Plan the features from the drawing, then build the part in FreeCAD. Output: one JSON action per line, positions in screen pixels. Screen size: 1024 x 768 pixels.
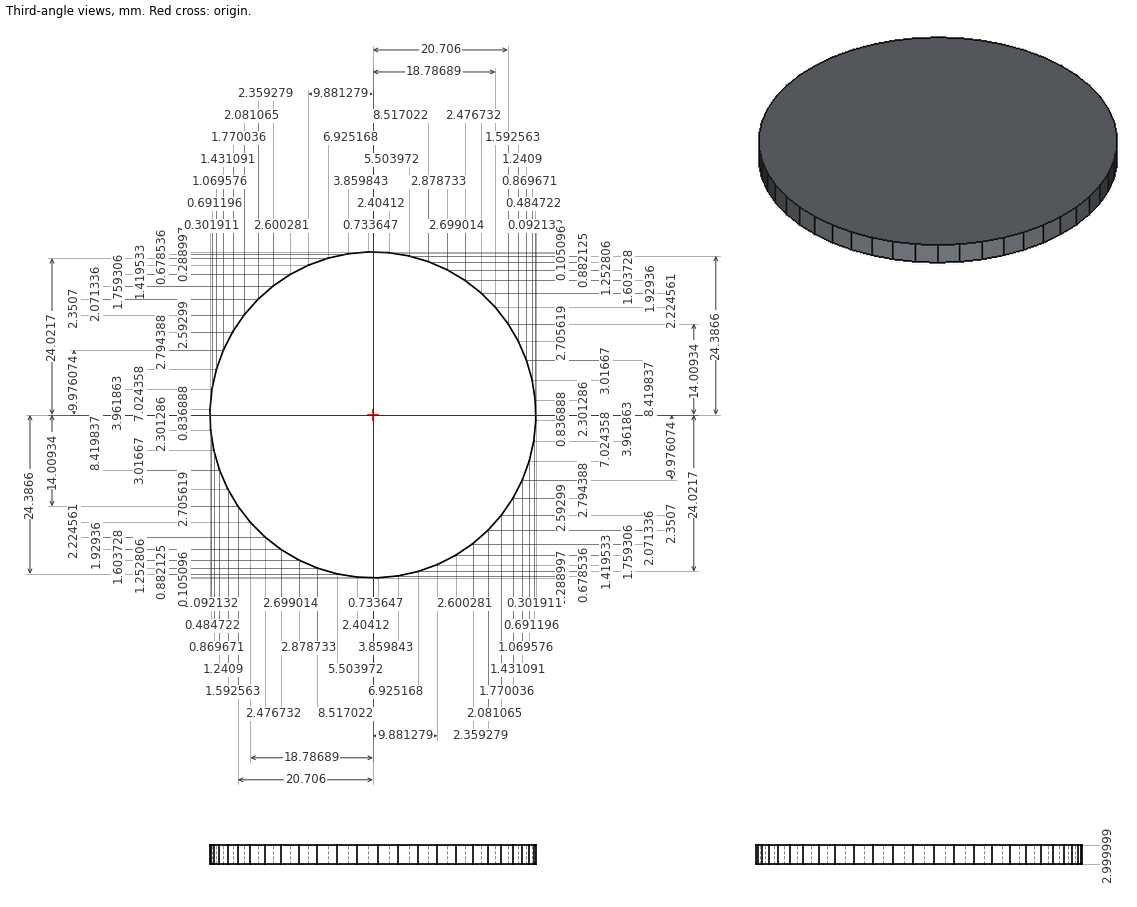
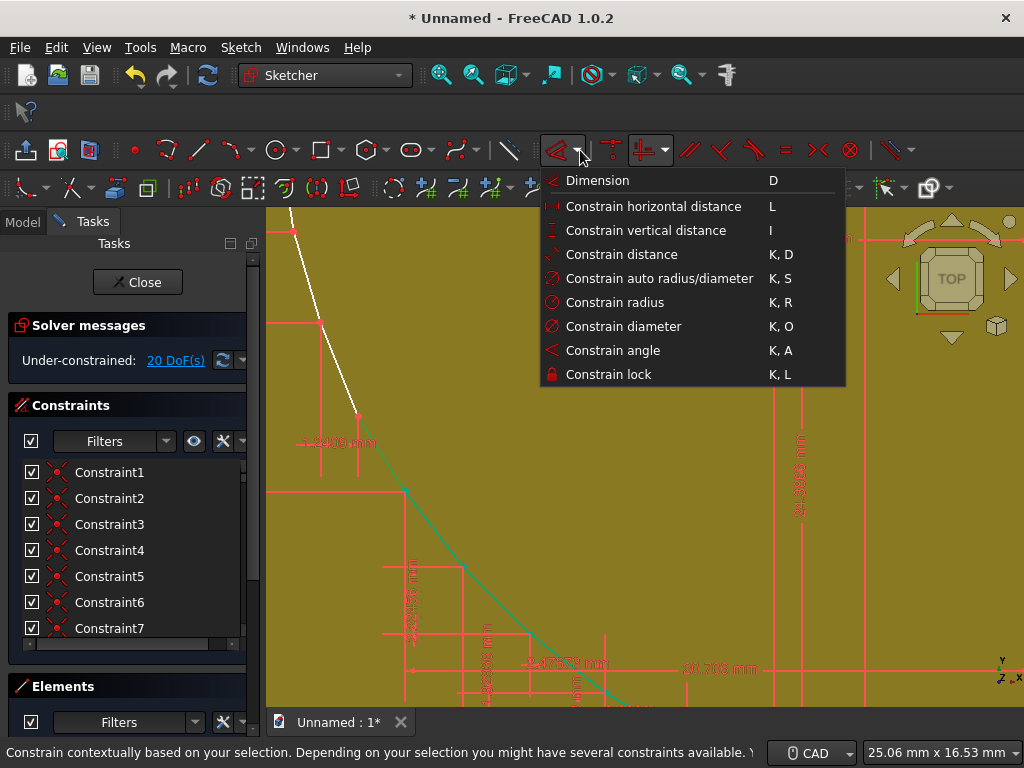
{"action": "left_click", "coordinate": [693, 206]}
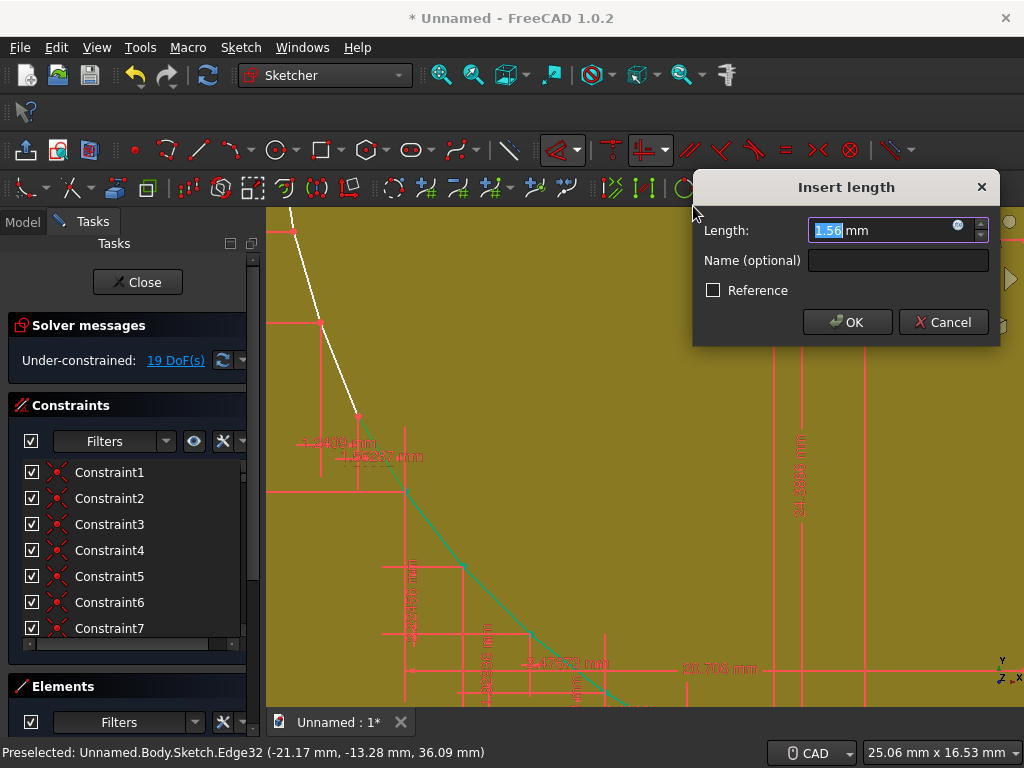
{"action": "type", "text": "1.592563"}
{"action": "key", "text": "Return"}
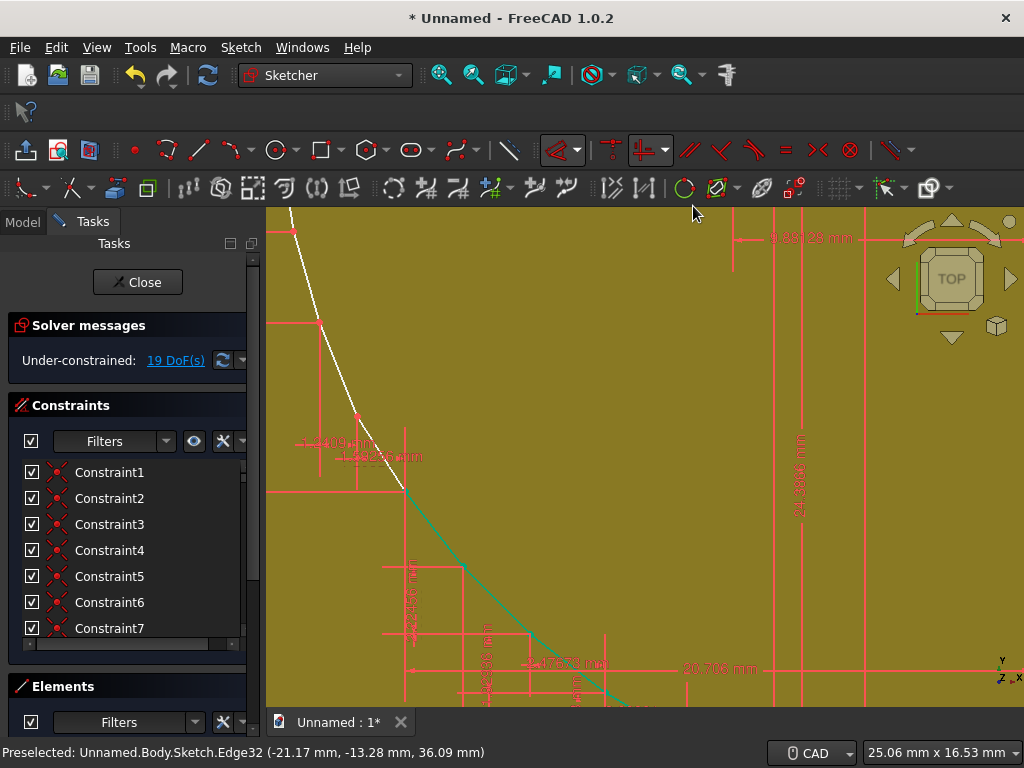
{"action": "left_click", "coordinate": [391, 469]}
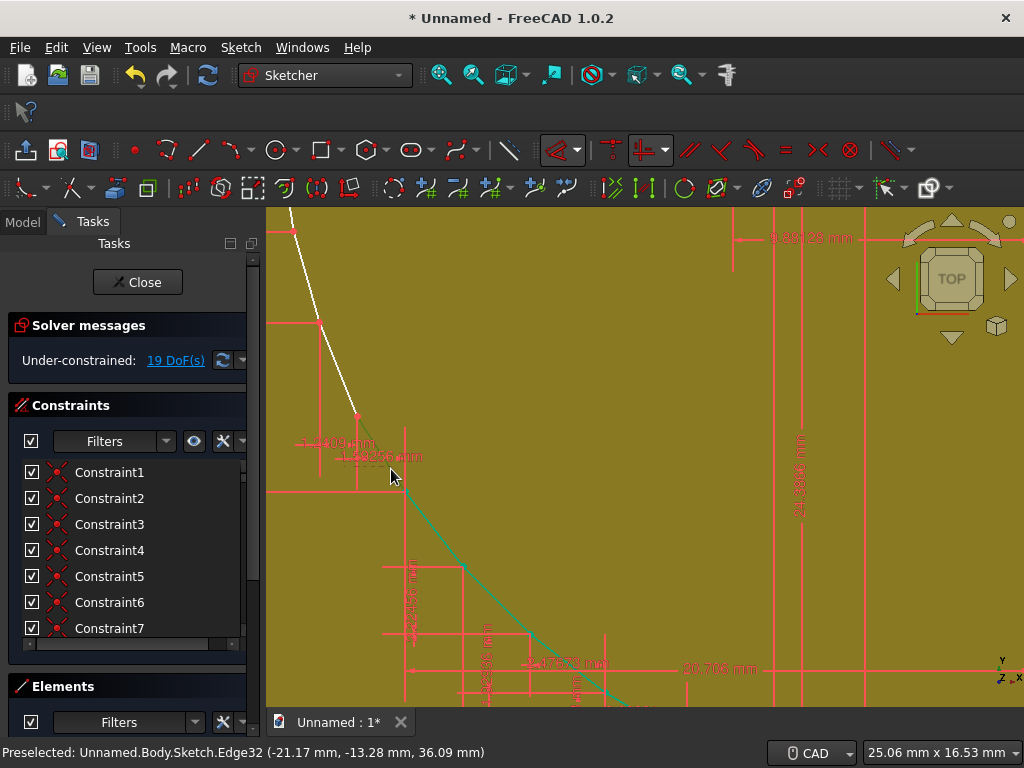
{"action": "left_click", "coordinate": [580, 150]}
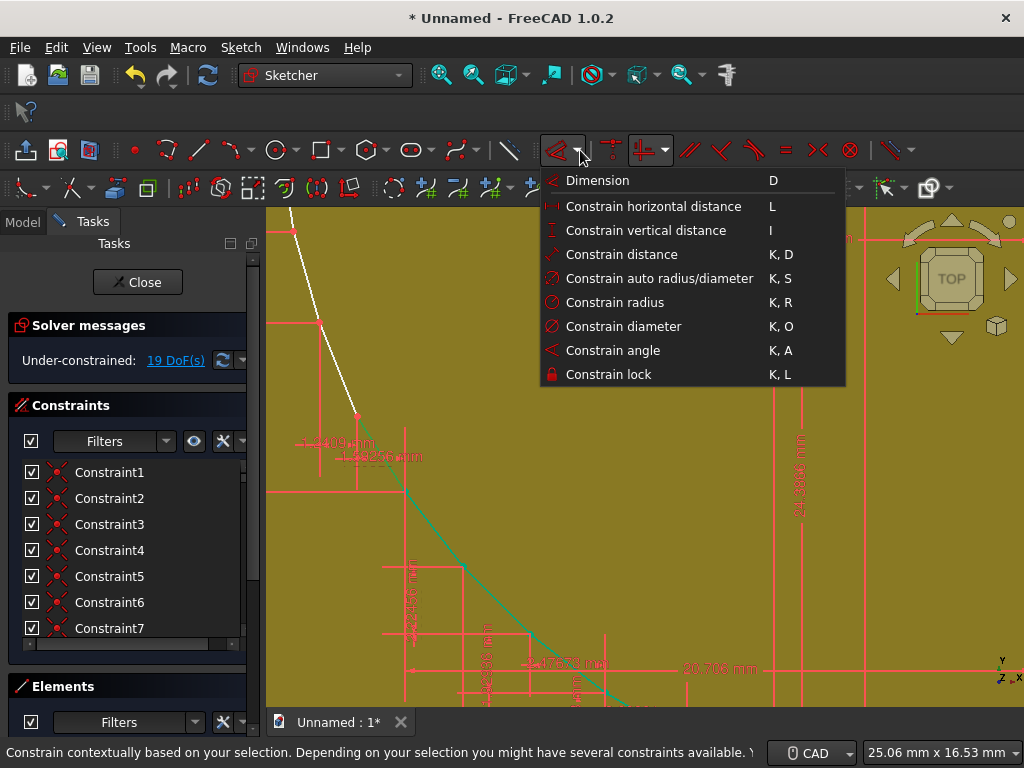
{"action": "left_click", "coordinate": [693, 230]}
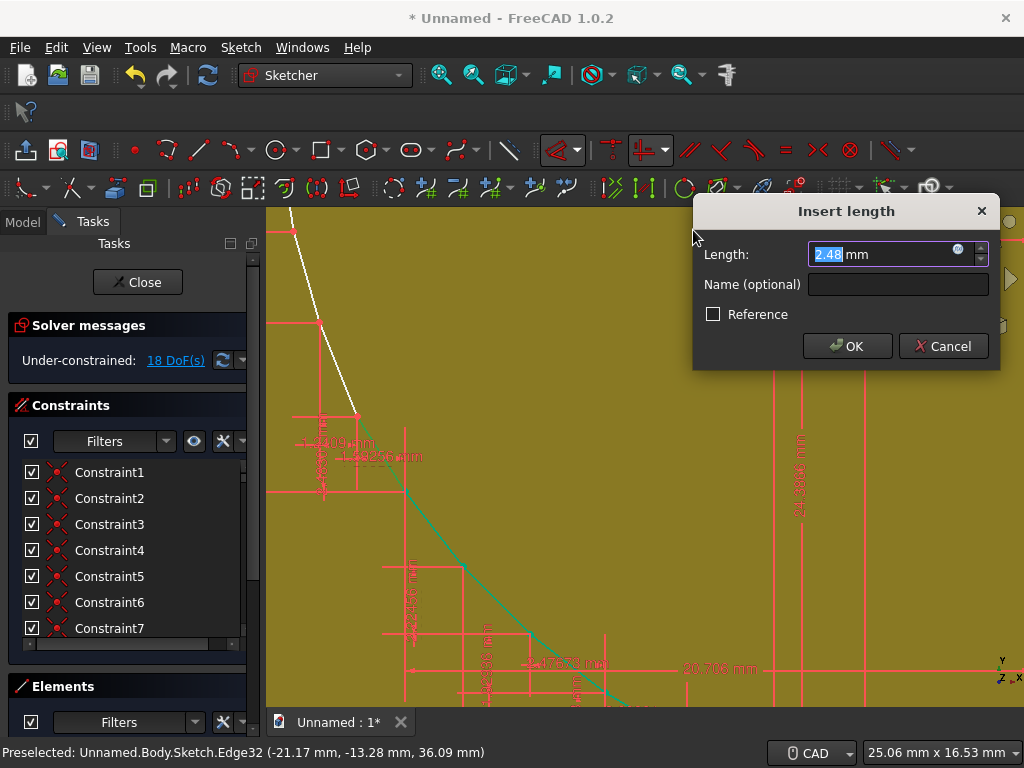
{"action": "type", "text": "2.705619"}
{"action": "key", "text": "Return"}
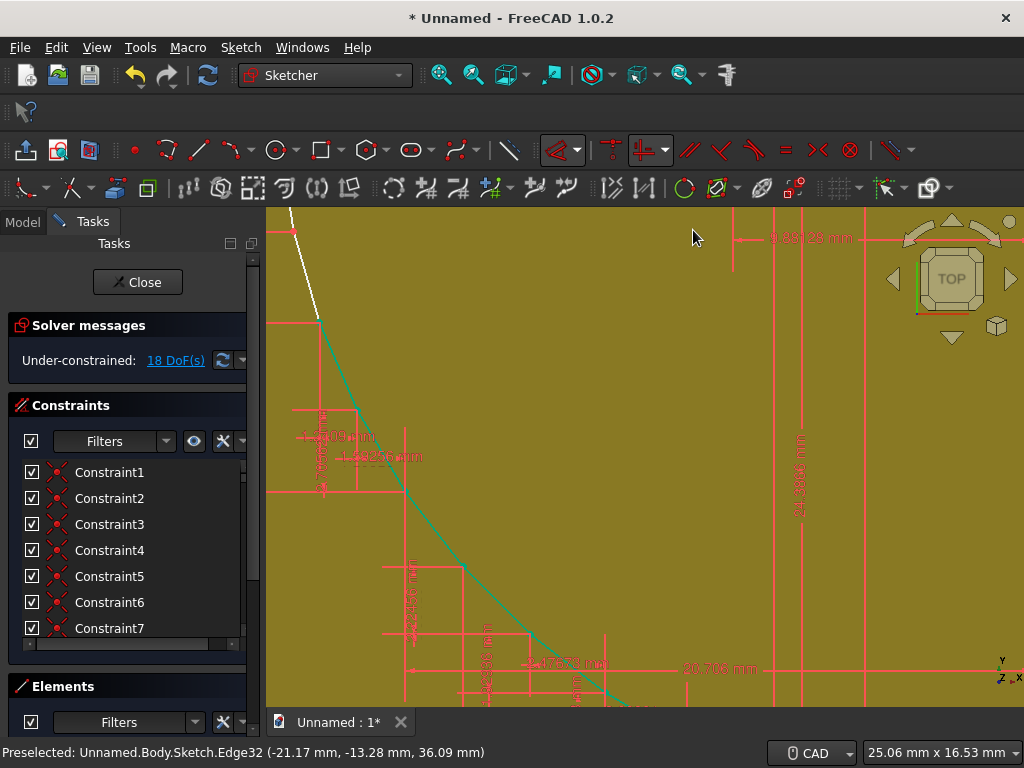
{"action": "scroll", "coordinate": [312, 295], "scroll_direction": "up", "scroll_amount": 3}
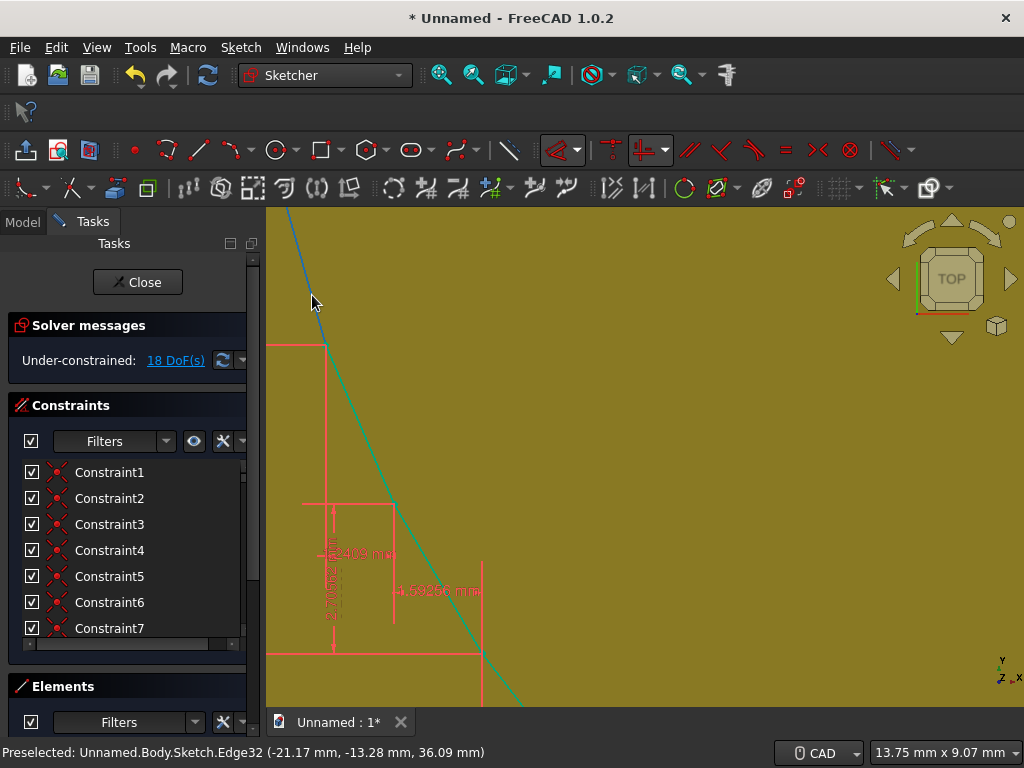
{"action": "left_click", "coordinate": [312, 296]}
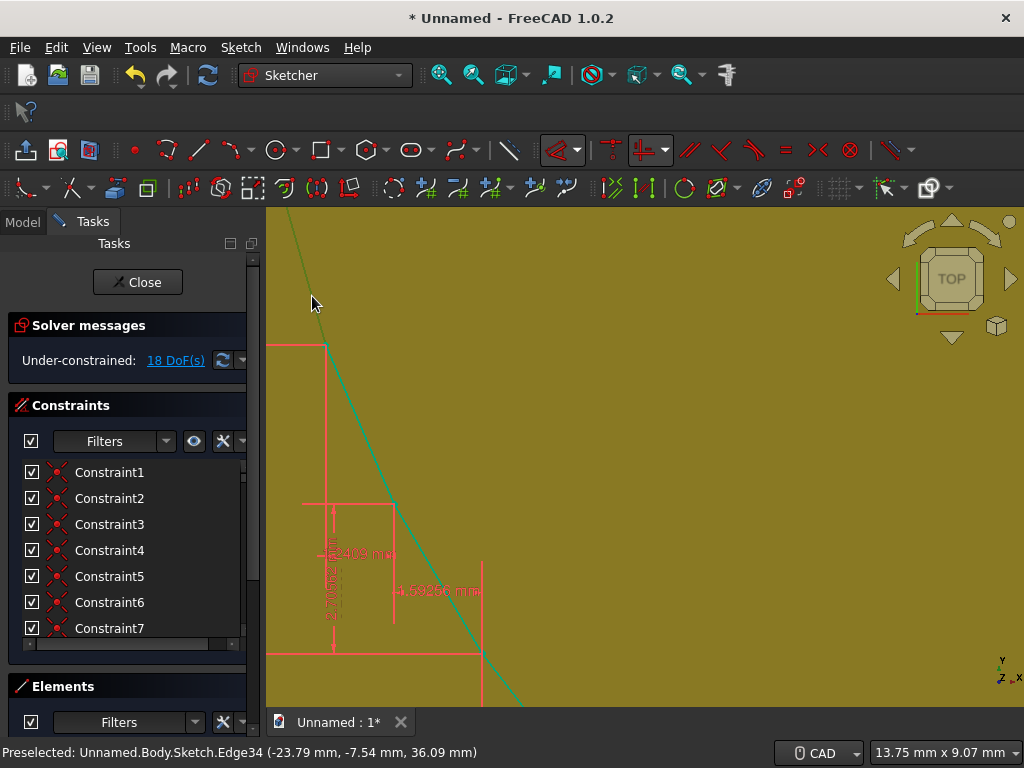
{"action": "key", "text": "l"}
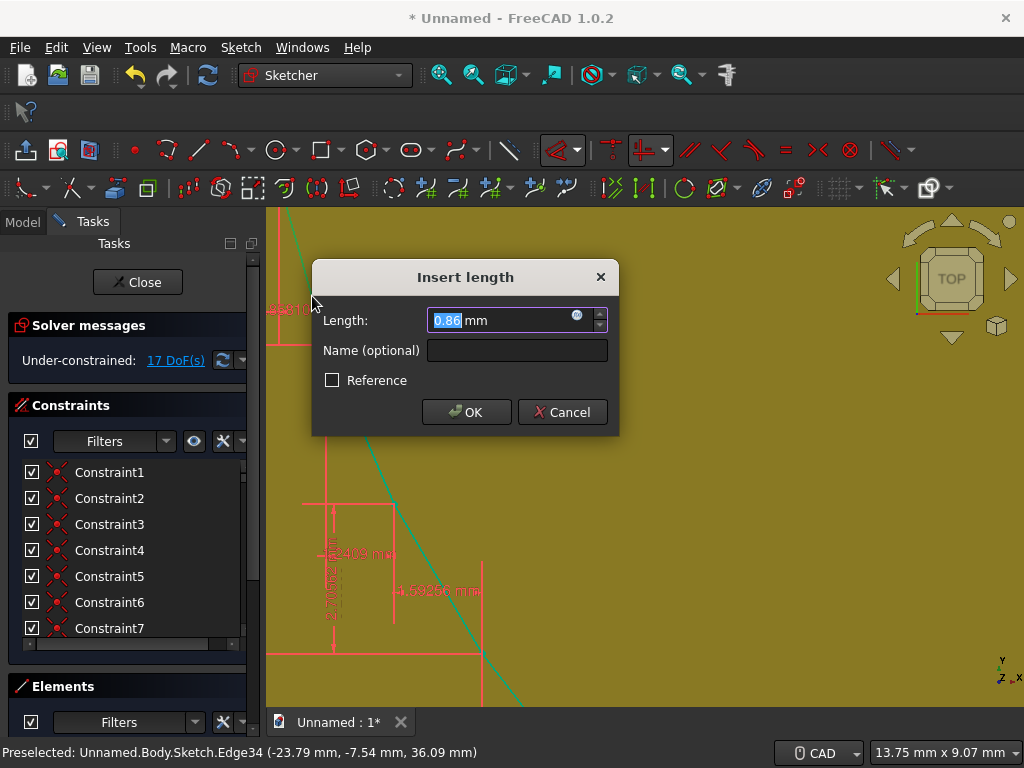
{"action": "type", "text": "0.869671"}
{"action": "key", "text": "Return"}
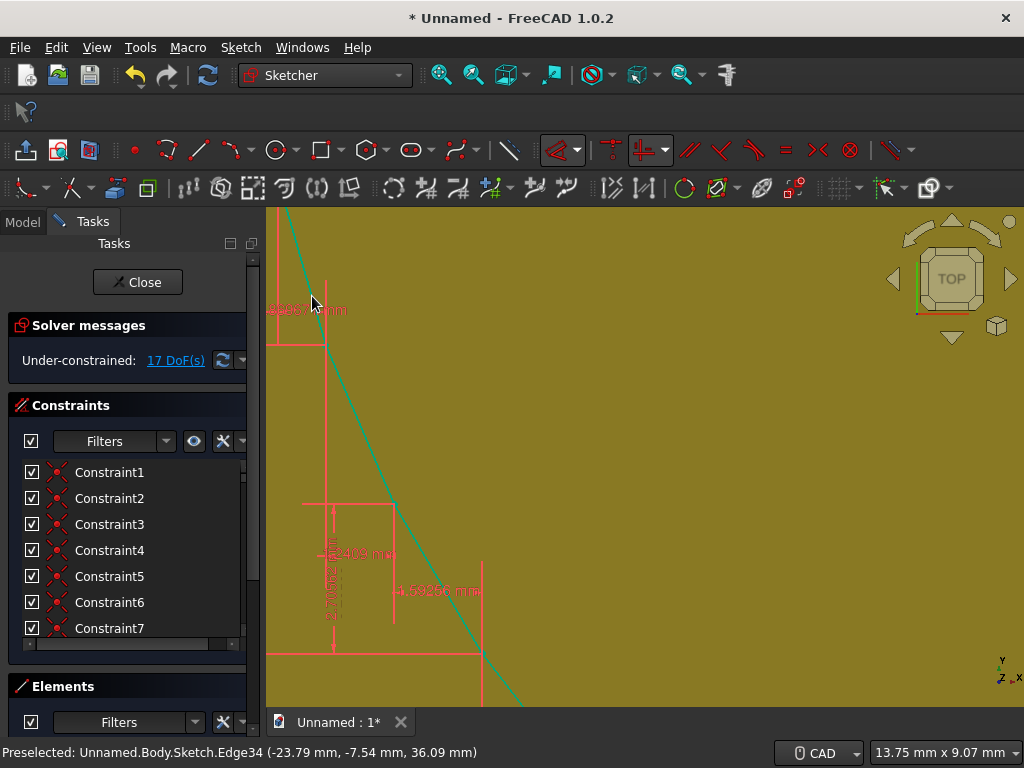
{"action": "scroll", "coordinate": [446, 529], "scroll_direction": "down", "scroll_amount": 11}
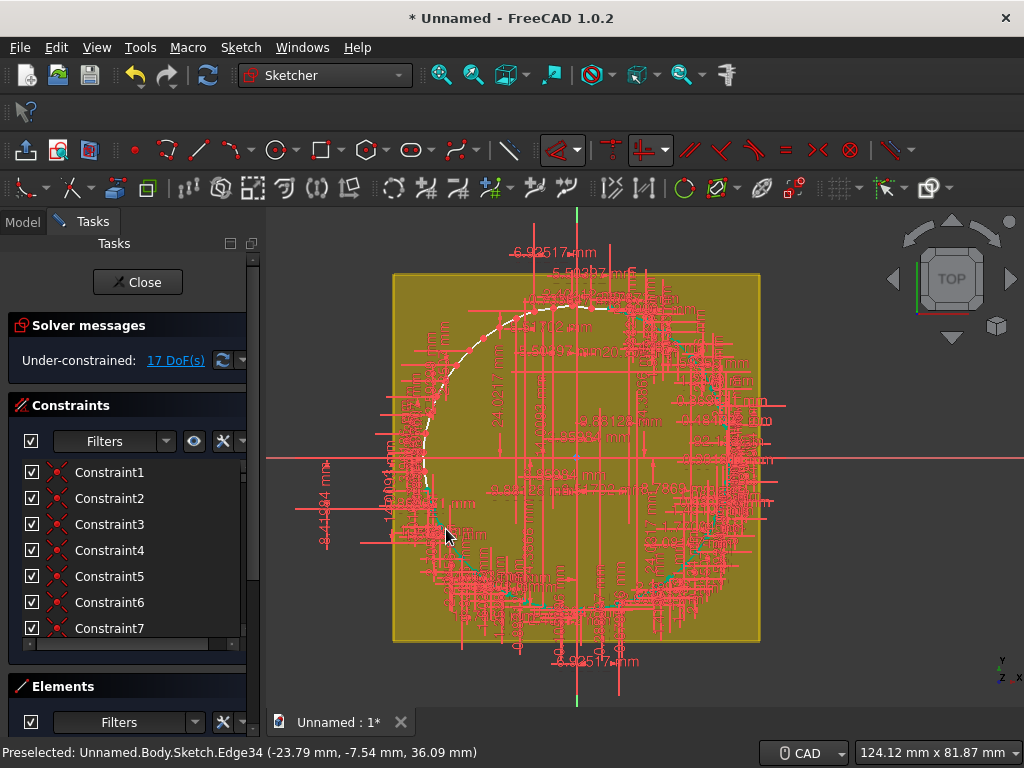
{"action": "scroll", "coordinate": [427, 485], "scroll_direction": "up", "scroll_amount": 13}